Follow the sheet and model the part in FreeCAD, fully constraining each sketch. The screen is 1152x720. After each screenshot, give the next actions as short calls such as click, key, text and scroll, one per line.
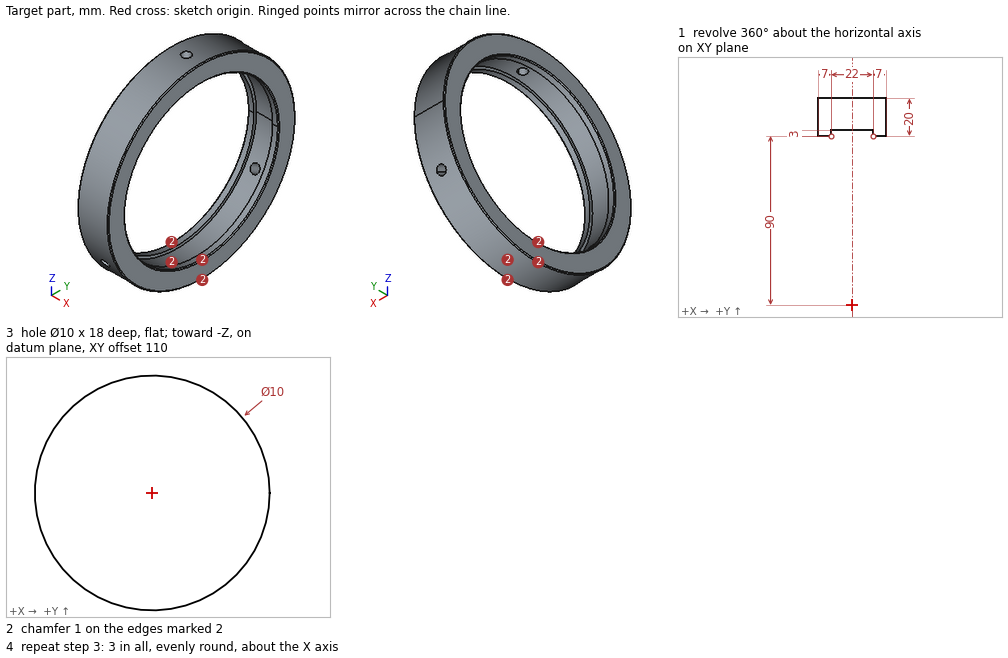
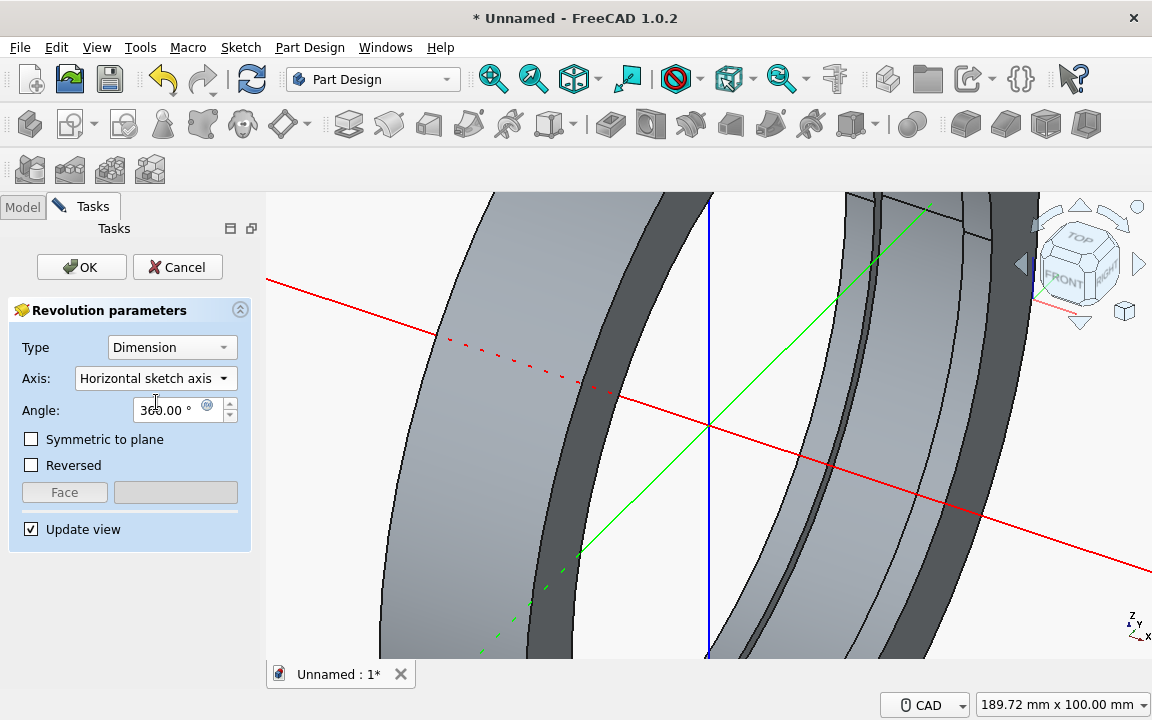
click(82, 267)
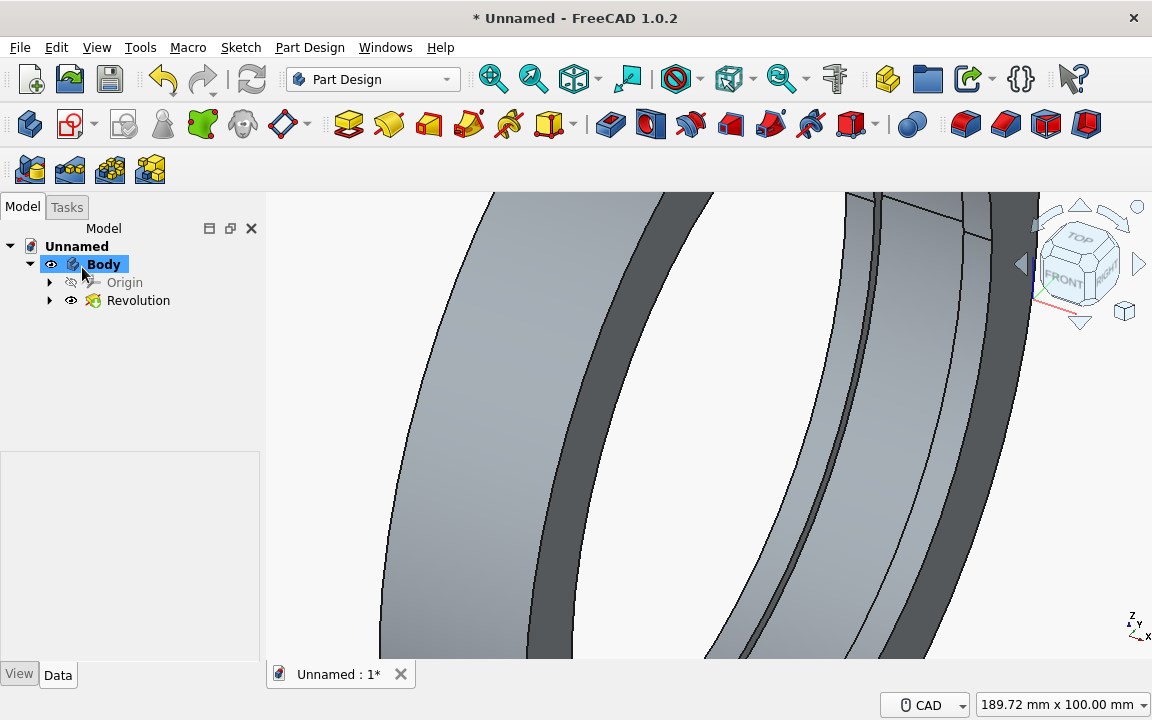
click(494, 80)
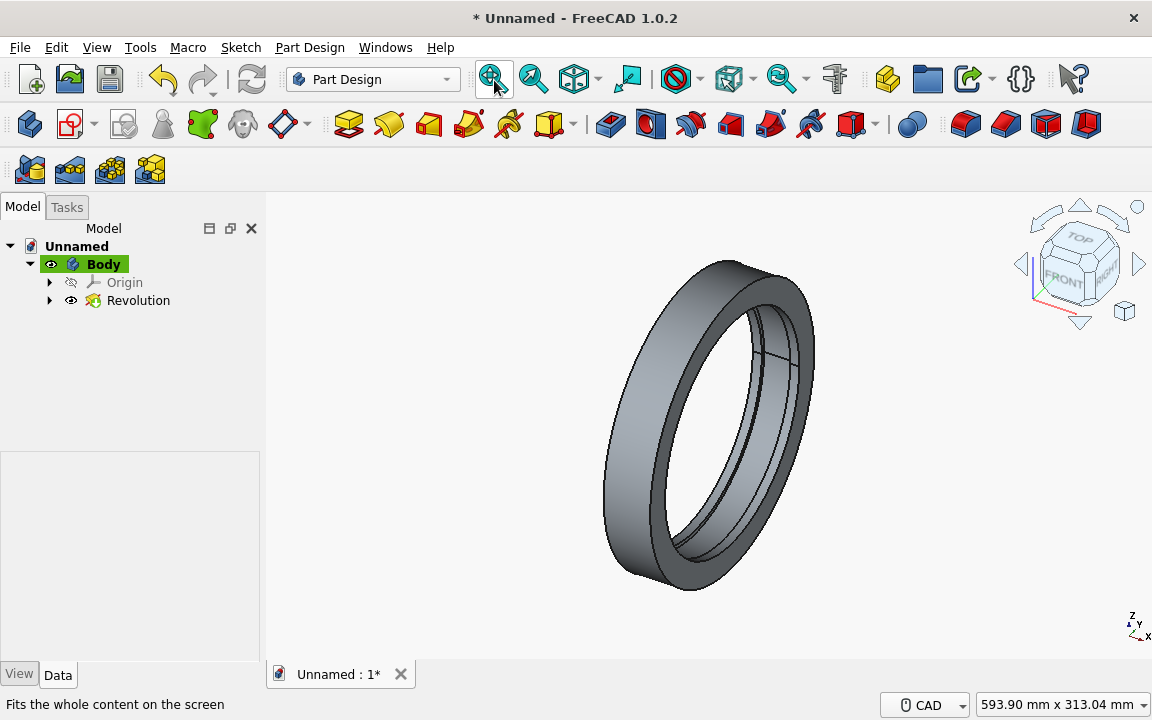
click(660, 314)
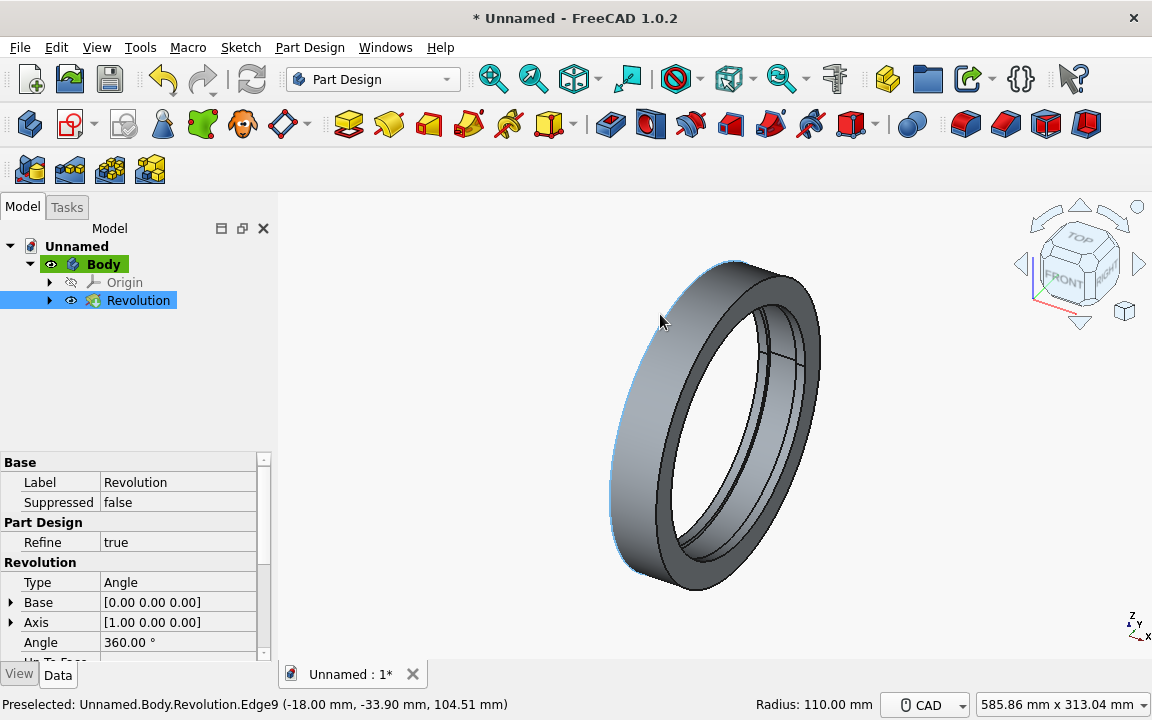
click(717, 557, ctrl)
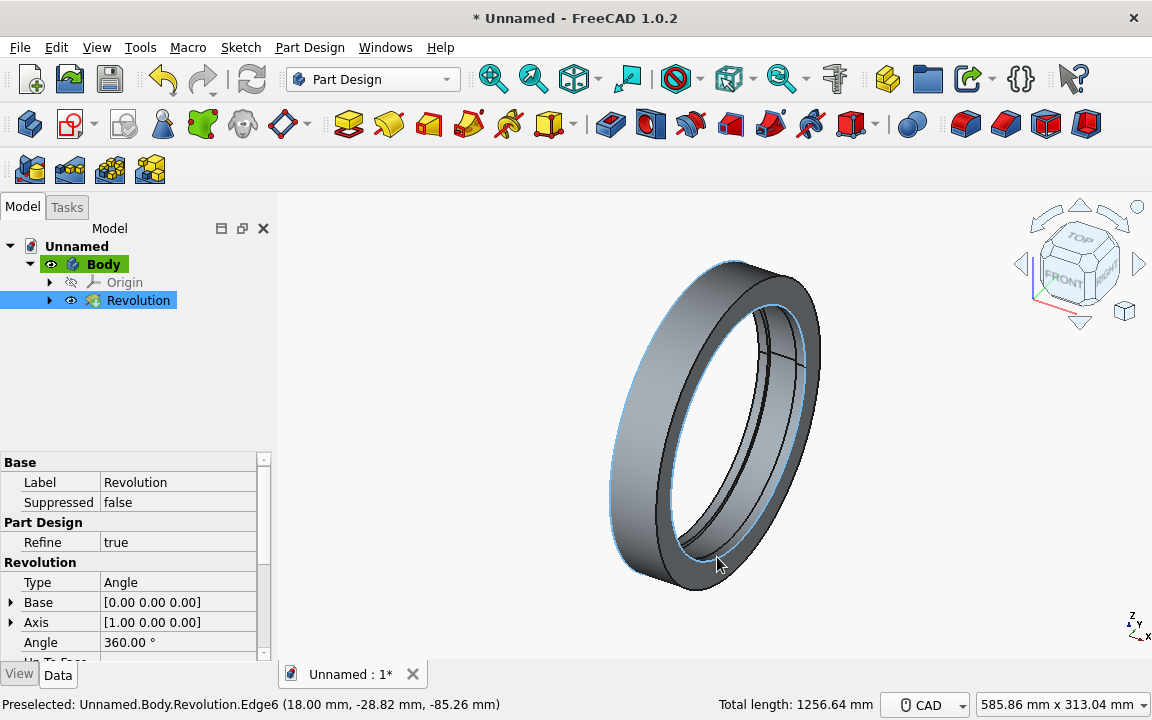
click(656, 514, ctrl)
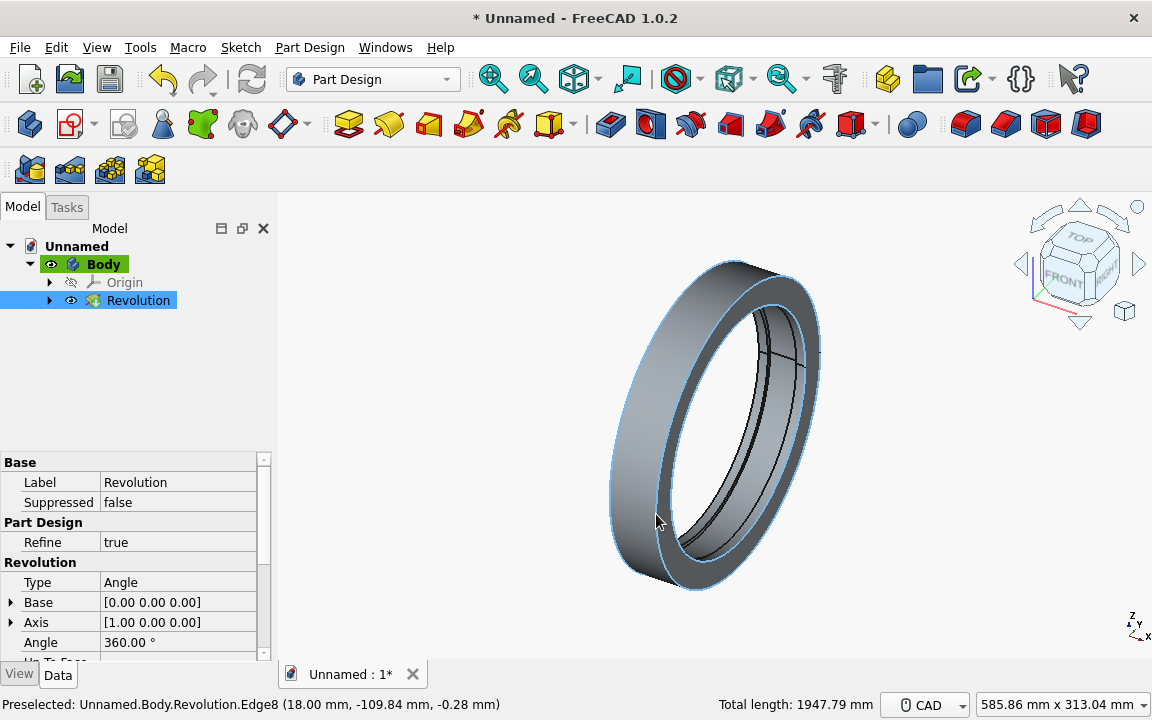
key(0)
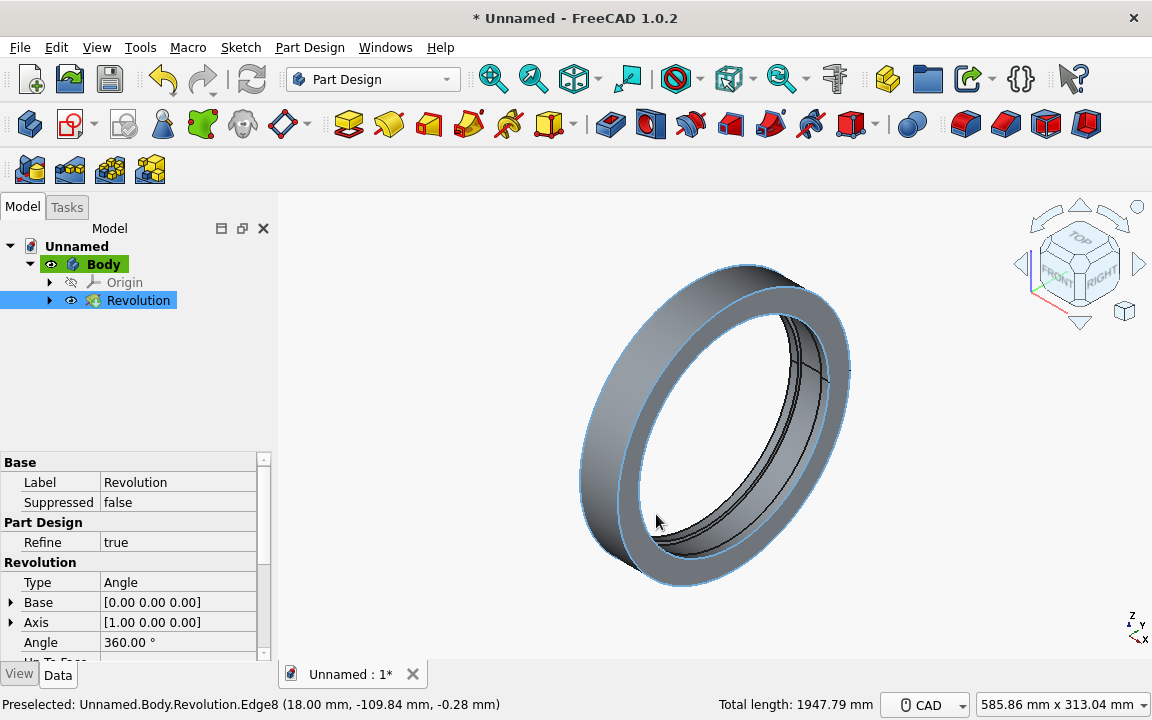
key(2)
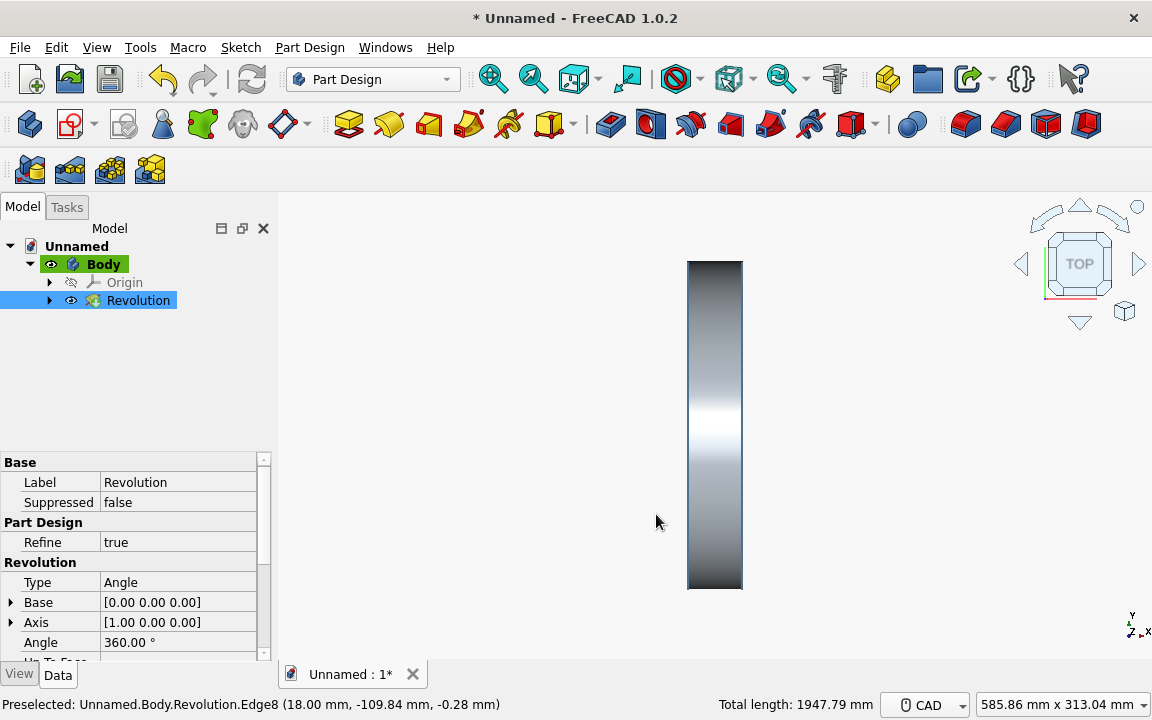
key(1)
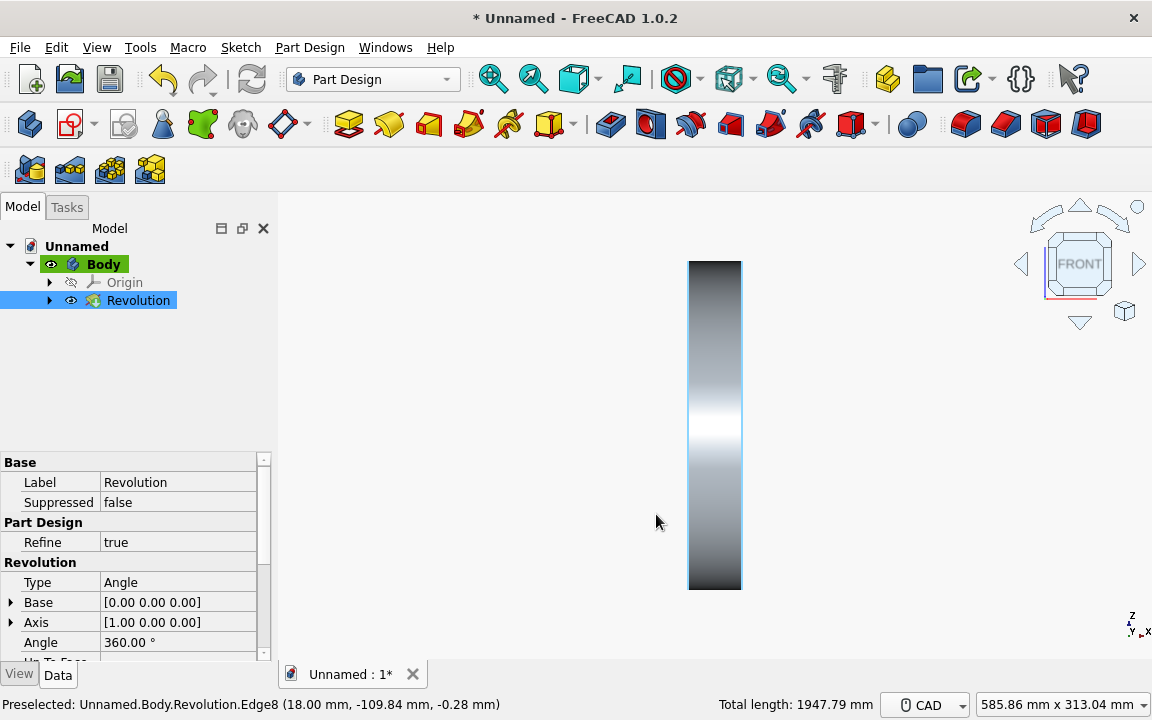
key(3)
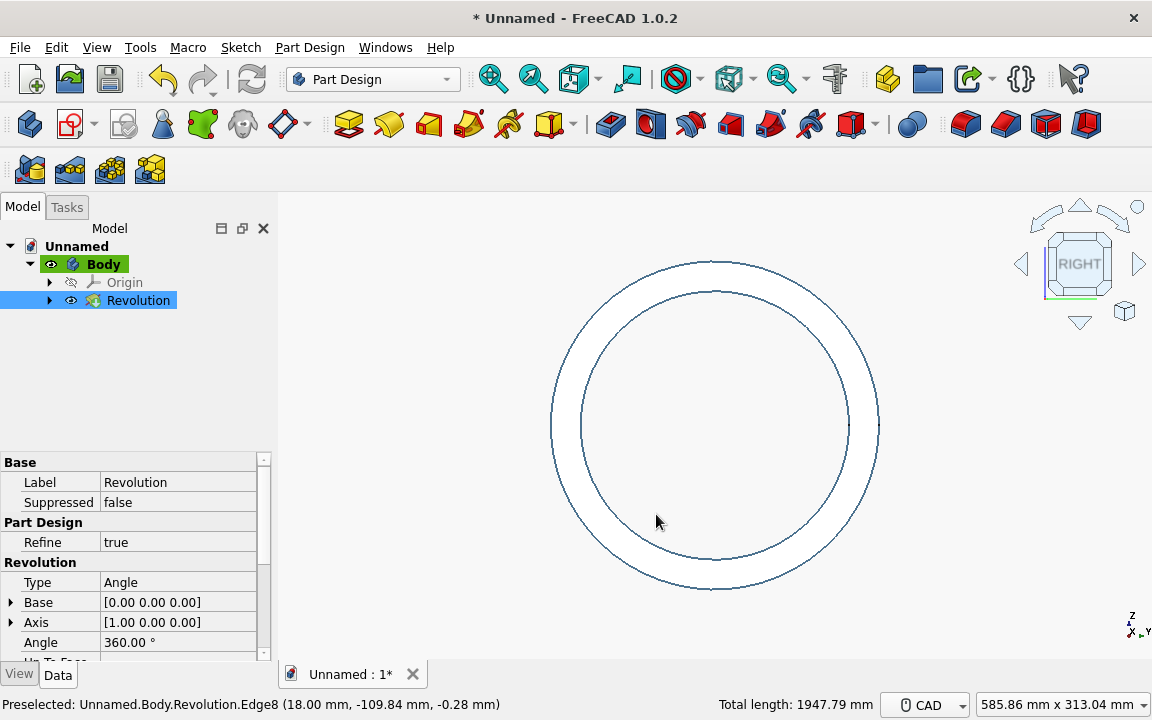
key(5)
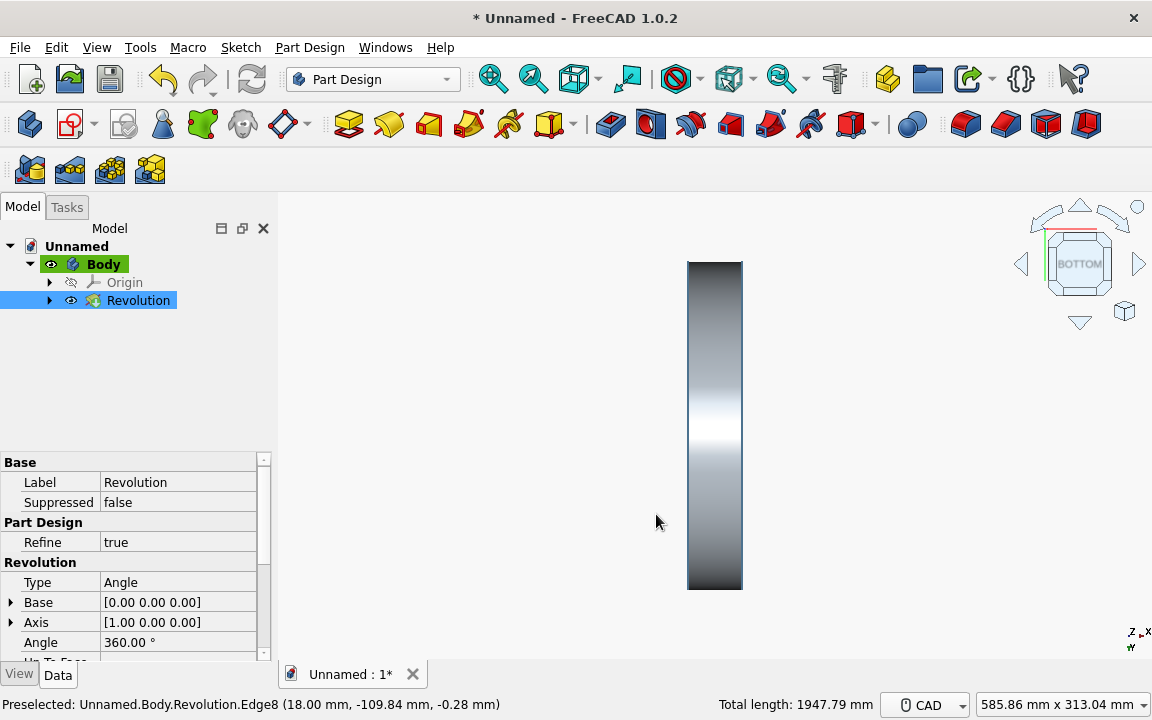
key(4)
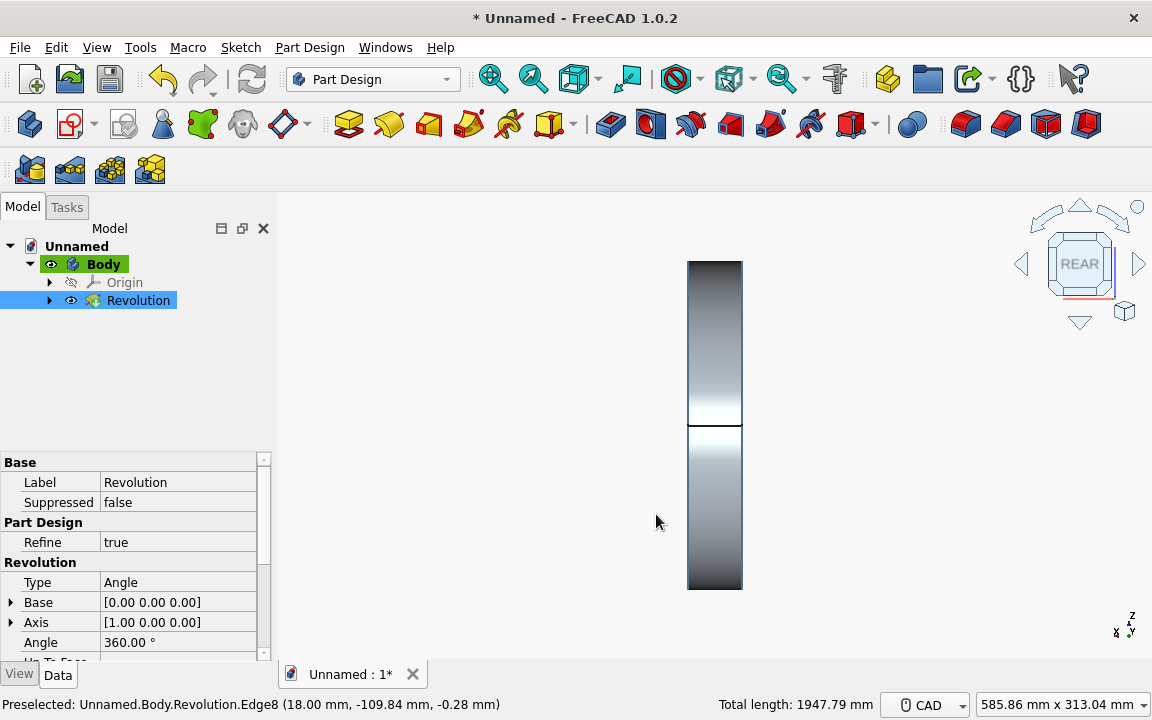
key(6)